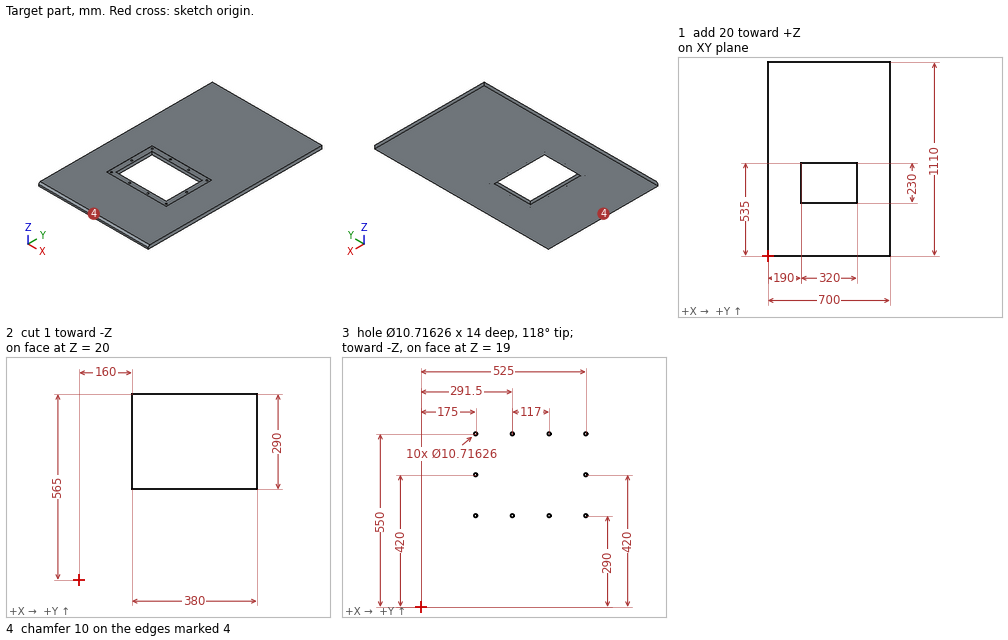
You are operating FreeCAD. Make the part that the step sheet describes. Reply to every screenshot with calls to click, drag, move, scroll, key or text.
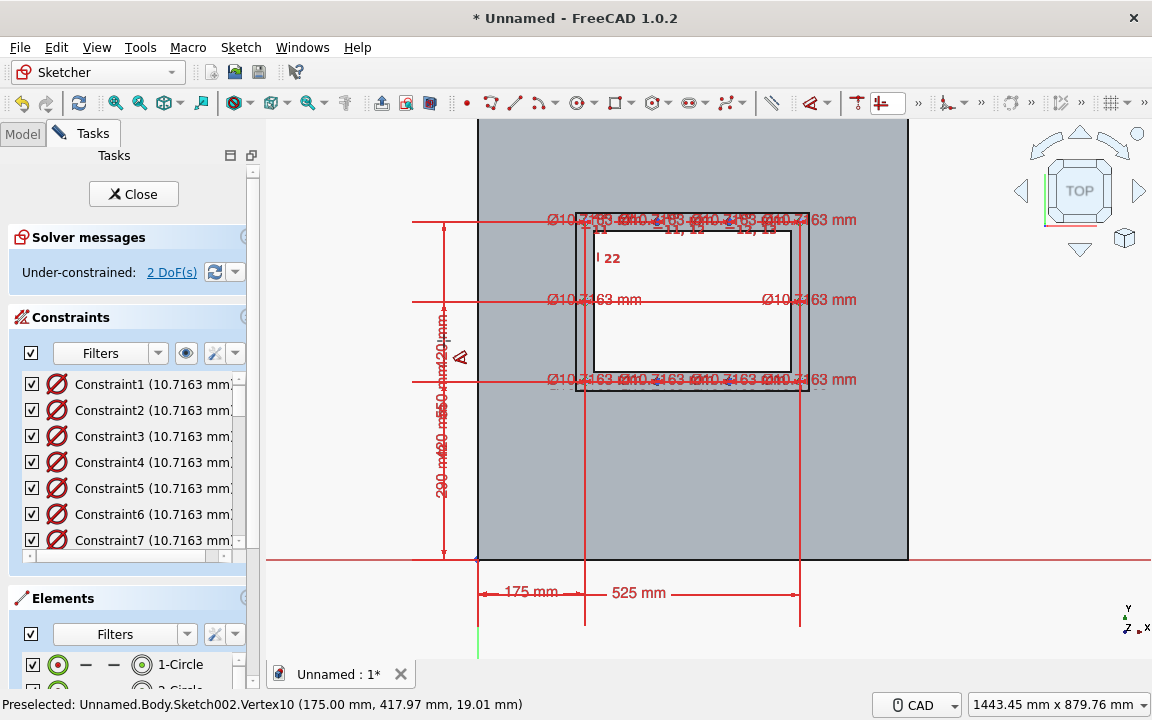
click(657, 222)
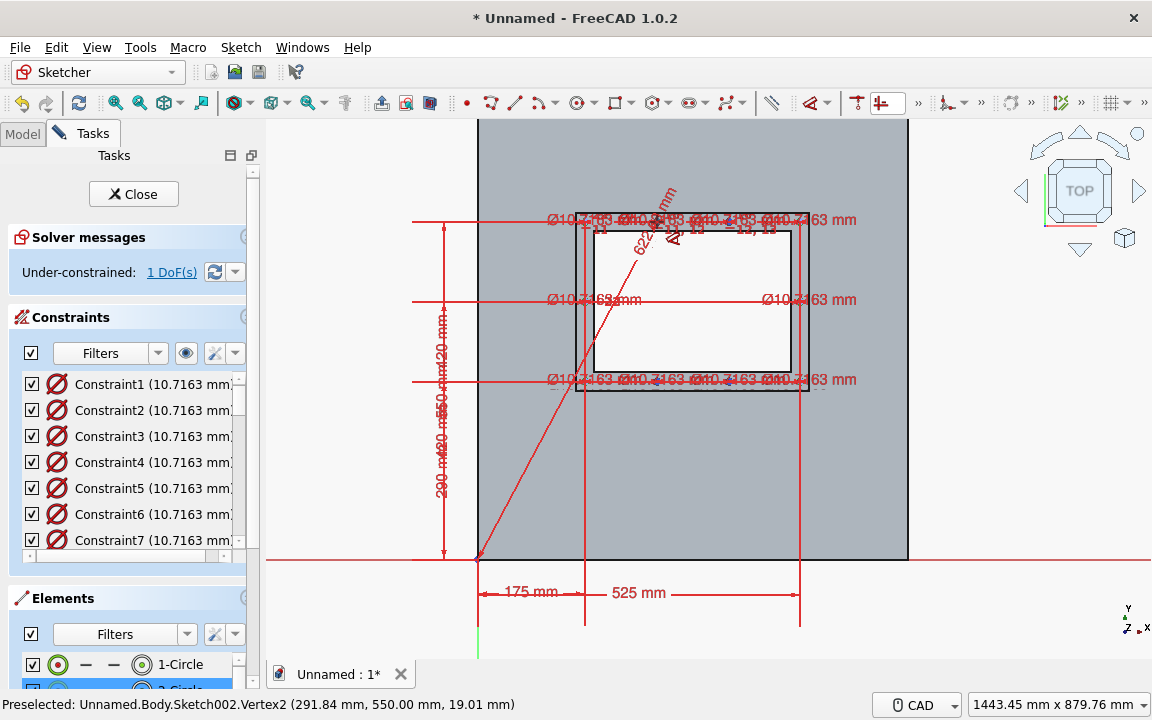
click(729, 222)
click(693, 188)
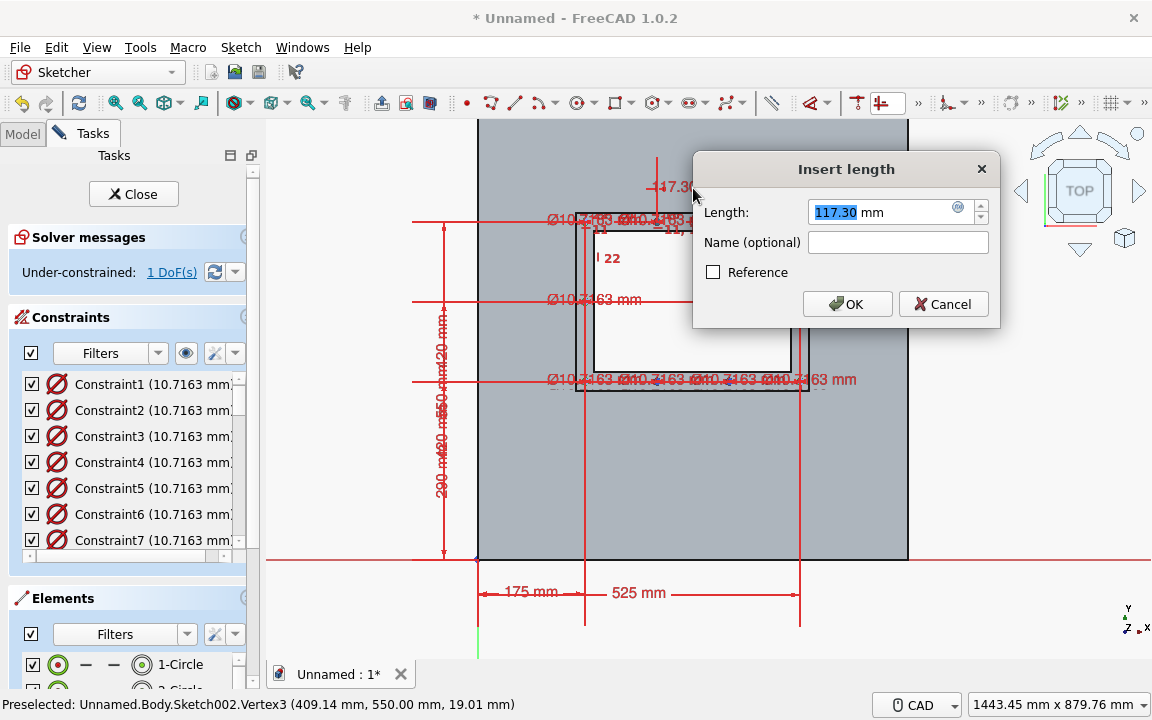
text(117)
key(Return)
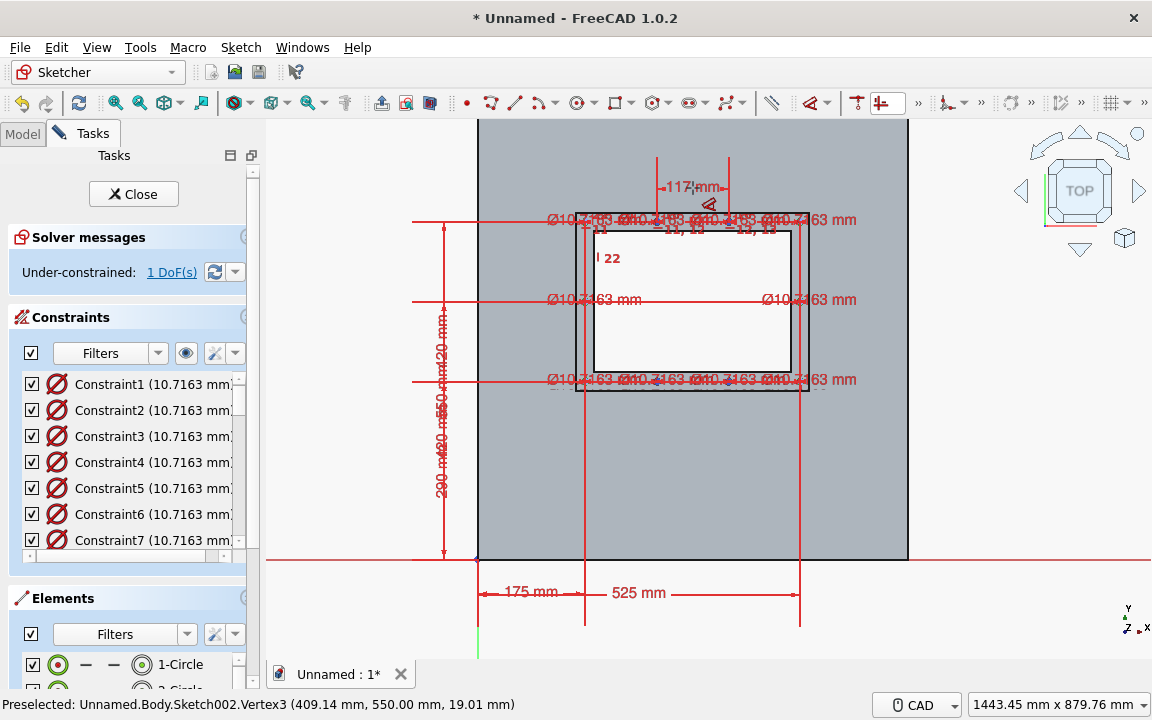
click(657, 222)
click(567, 188)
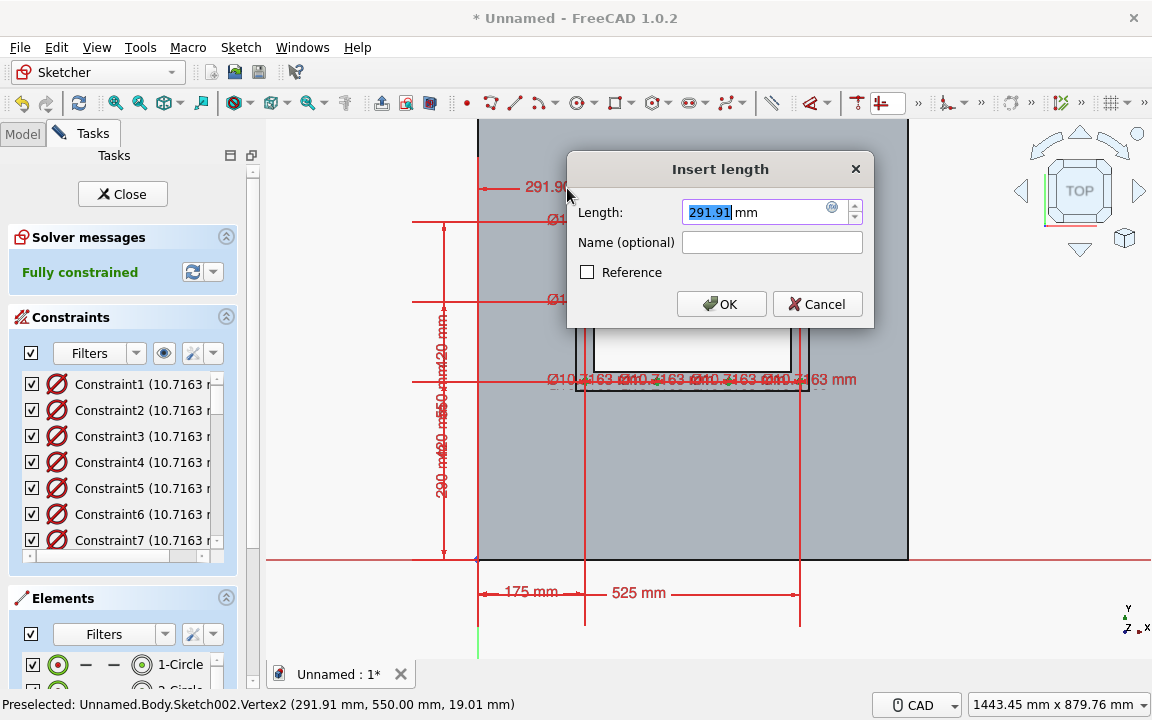
text(291.5)
key(Return)
key(Escape)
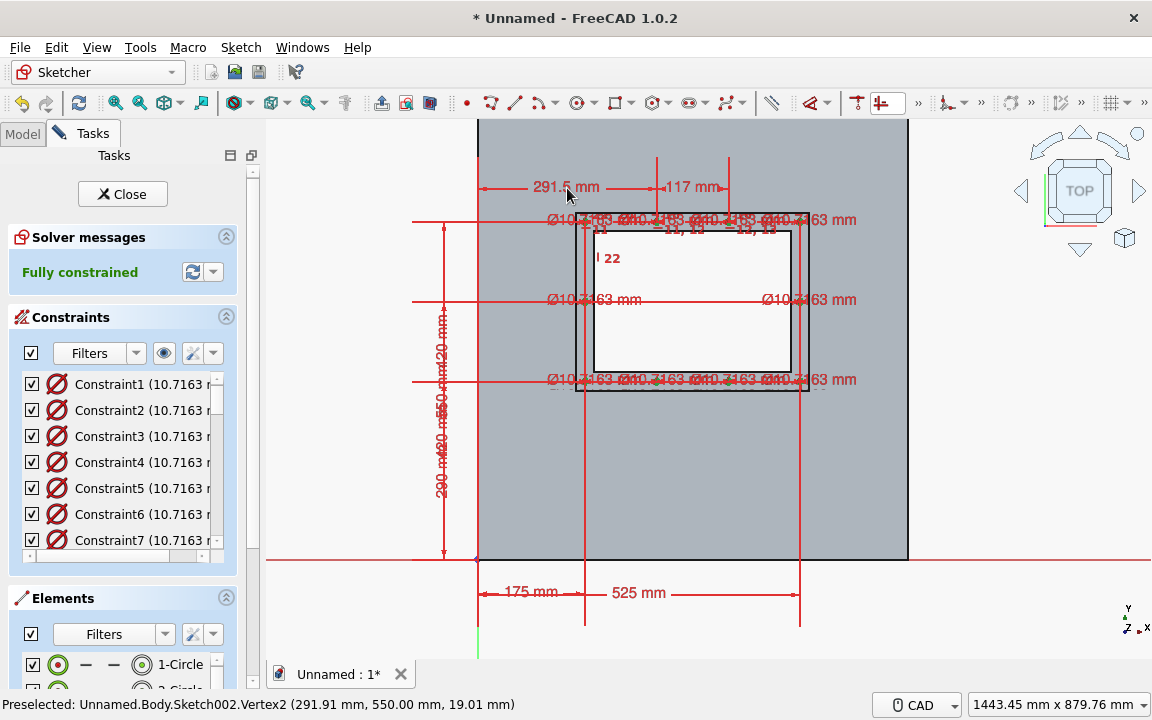
click(123, 194)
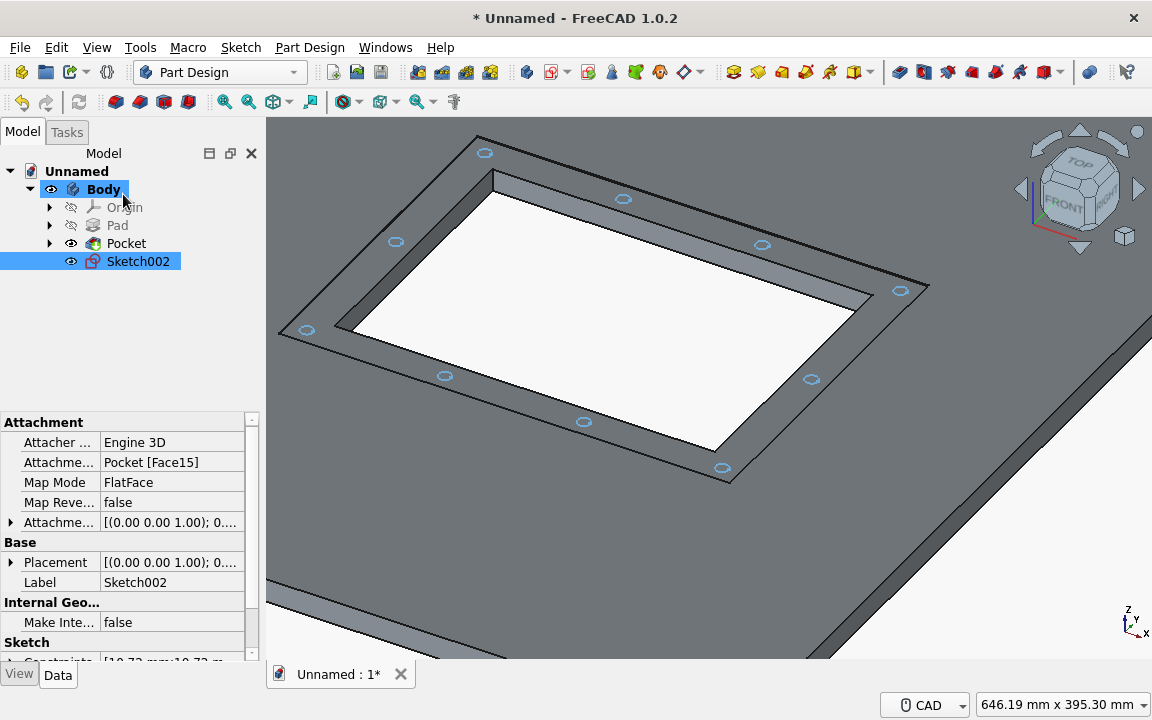
click(924, 72)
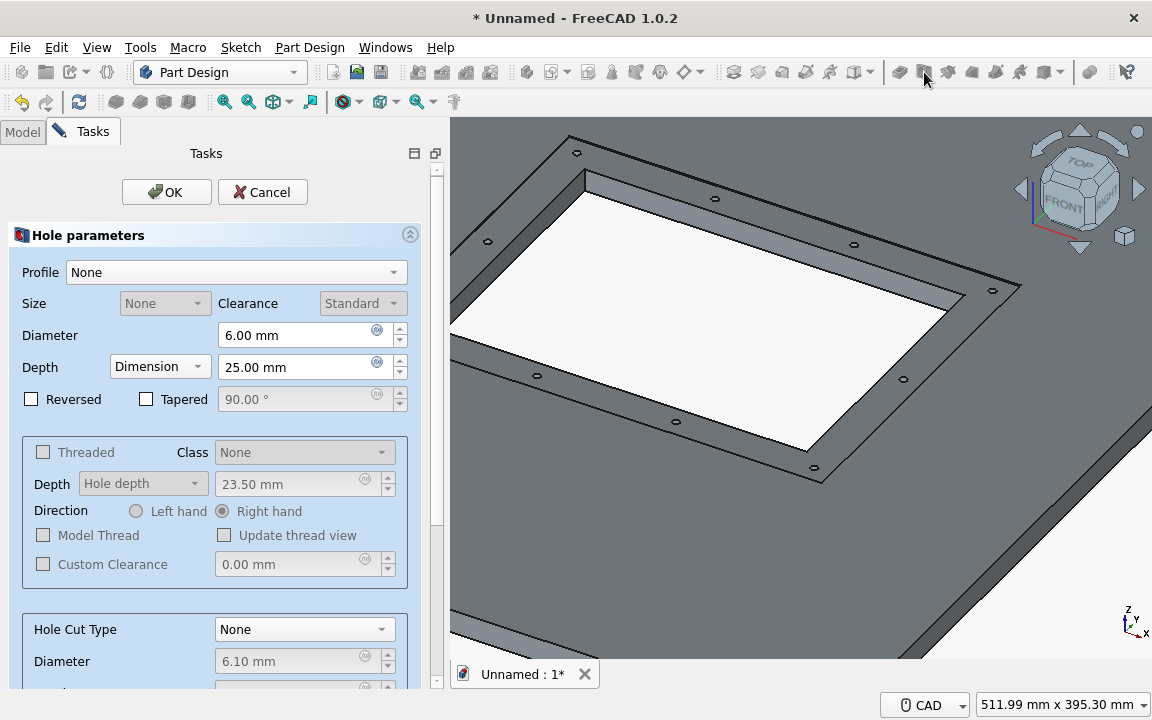
triple_click(305, 335)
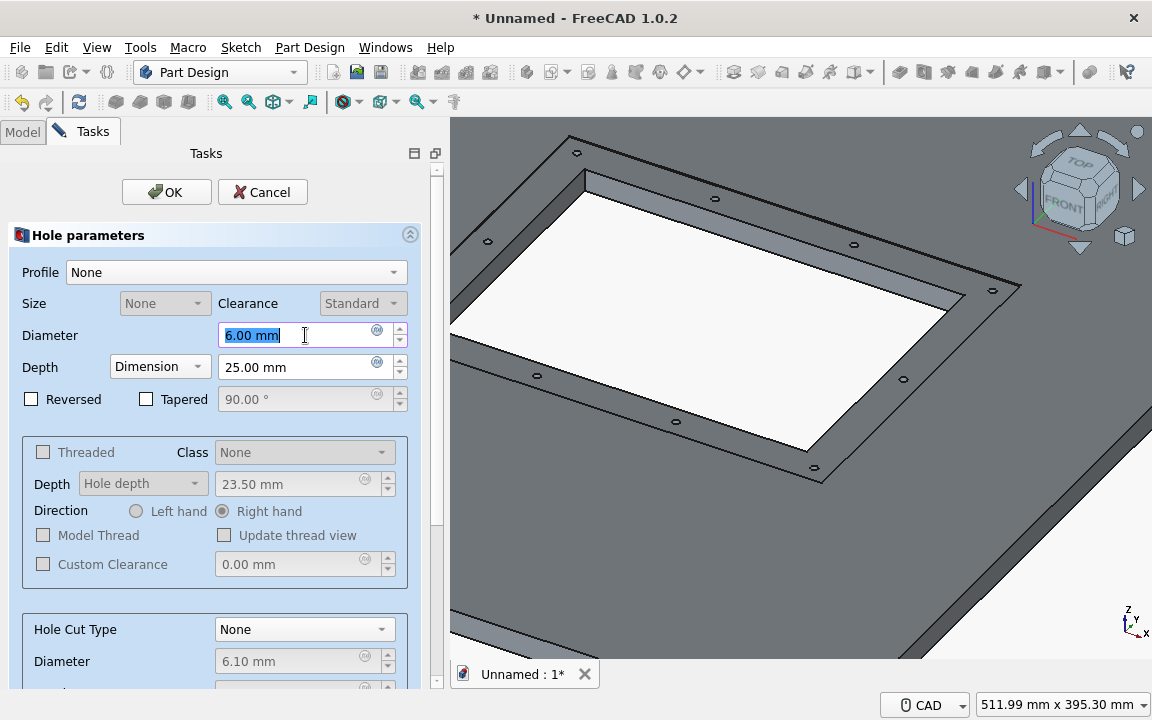
text(10.71626)
key(Tab)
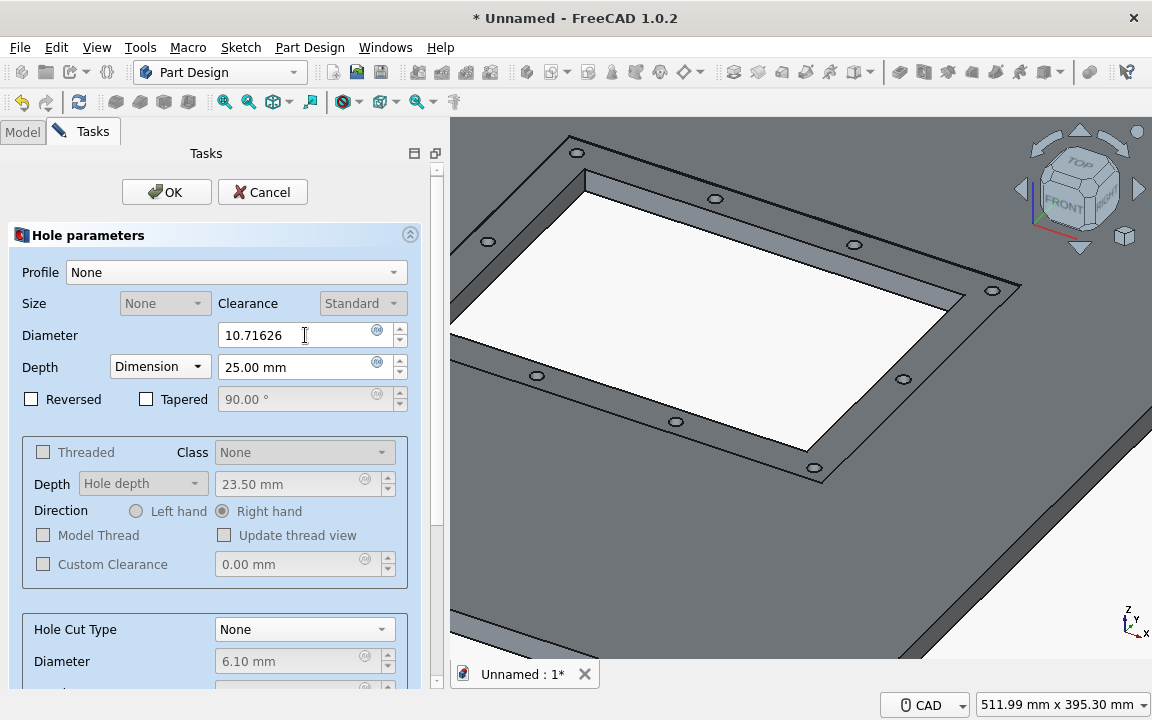
triple_click(305, 367)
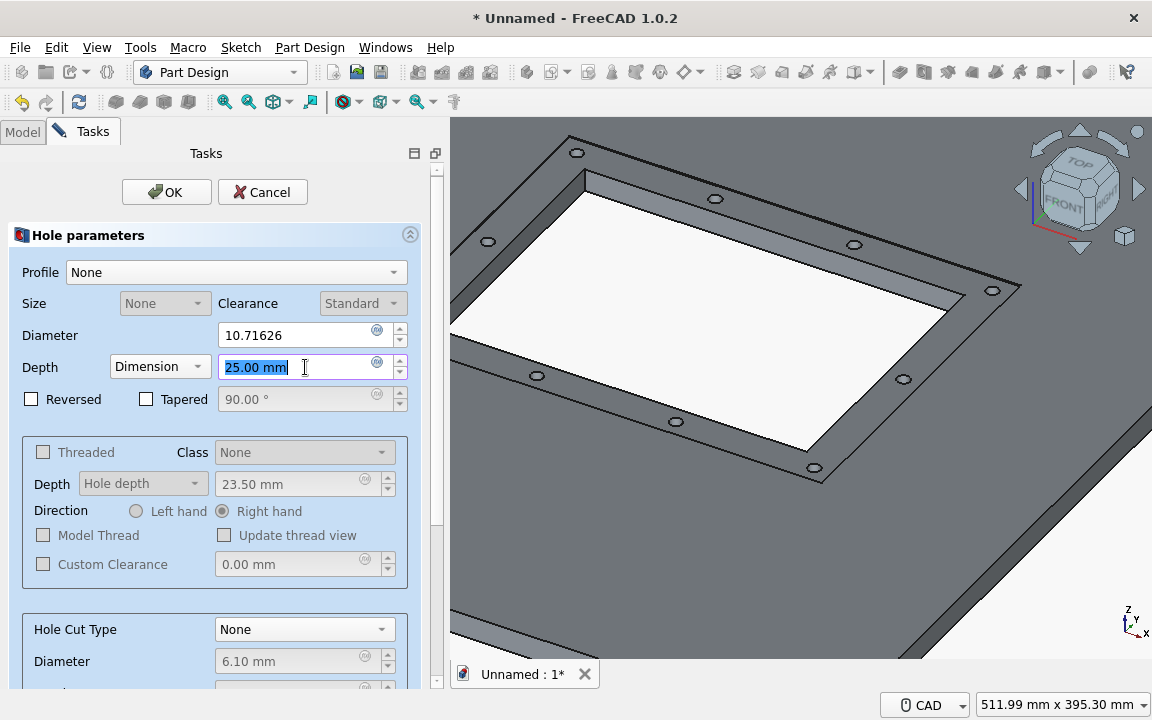
text(14)
key(Tab)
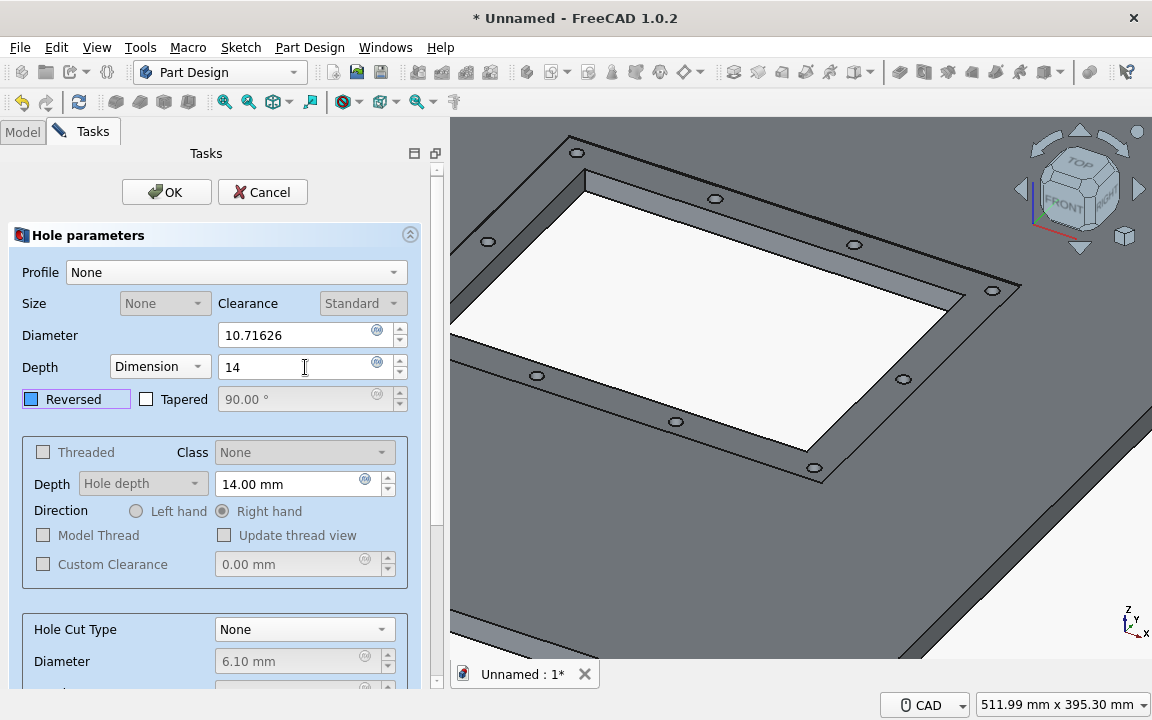
click(167, 192)